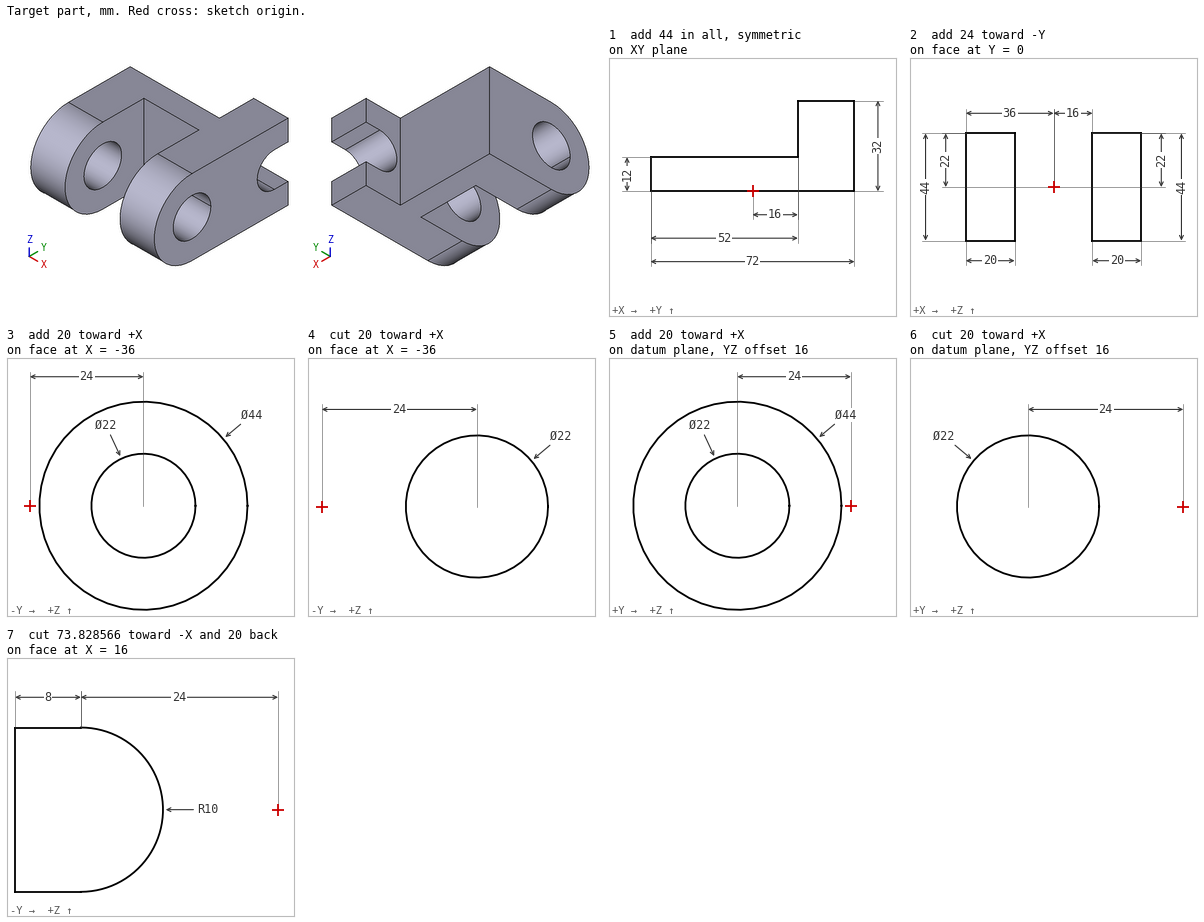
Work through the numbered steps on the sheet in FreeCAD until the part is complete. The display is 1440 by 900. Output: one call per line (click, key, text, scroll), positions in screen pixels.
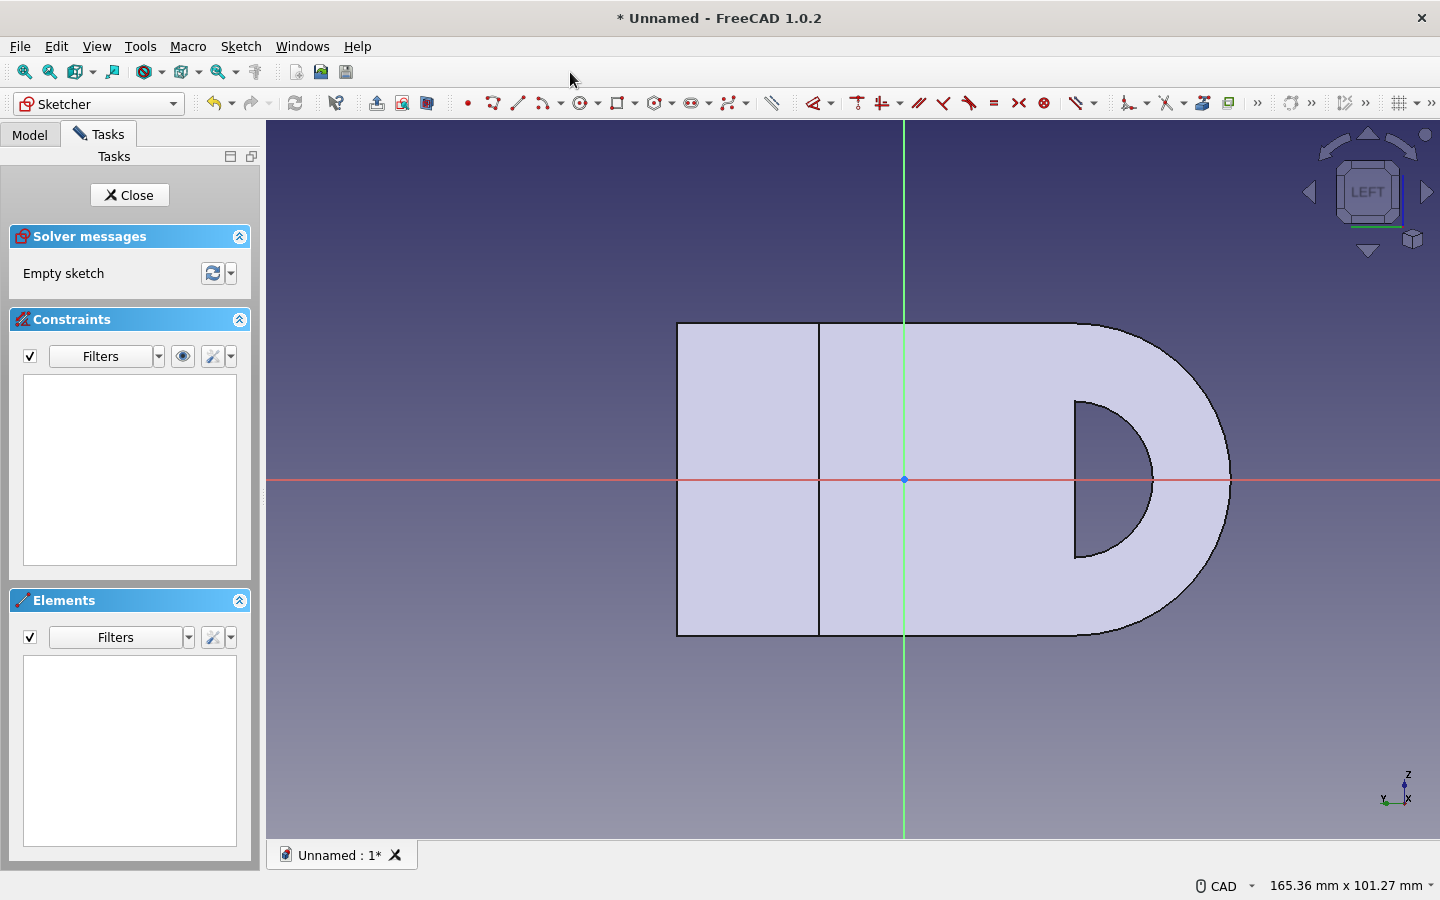
scroll(1171, 480, up, 5)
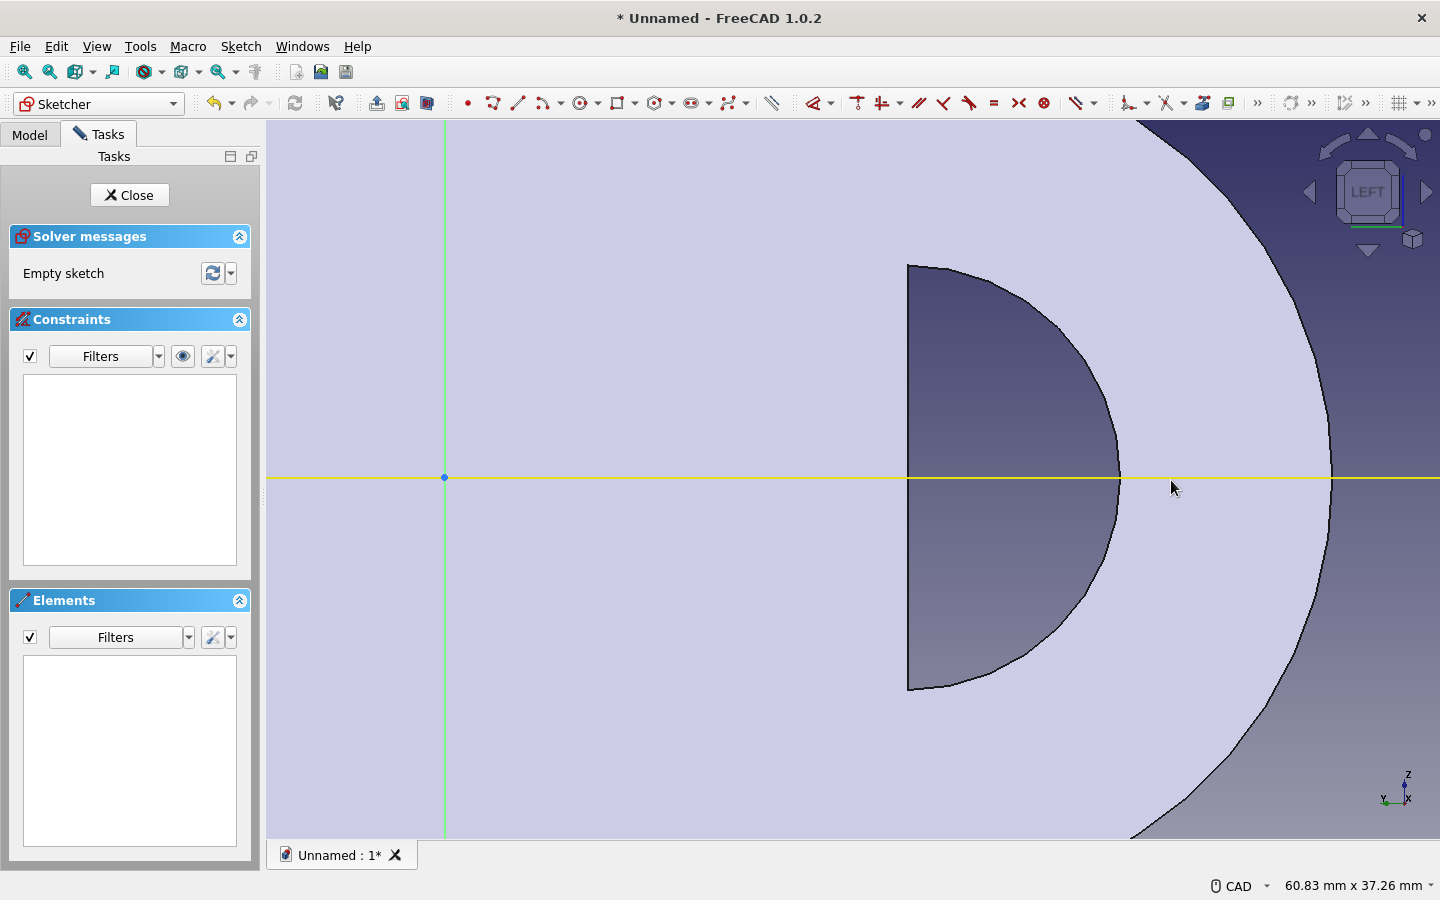
click(580, 104)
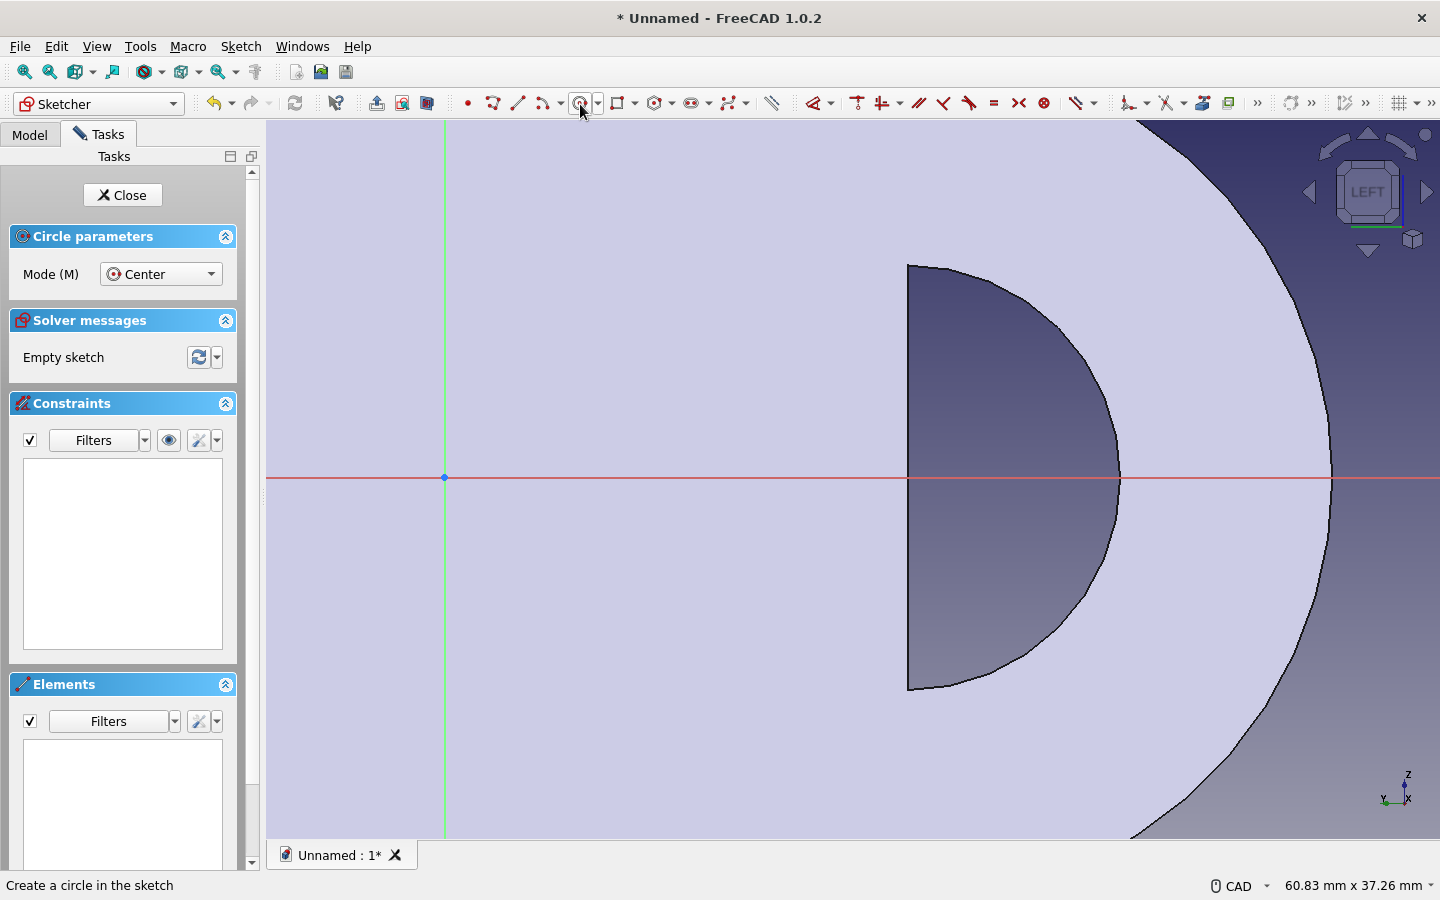
click(908, 478)
click(1058, 328)
key(Escape)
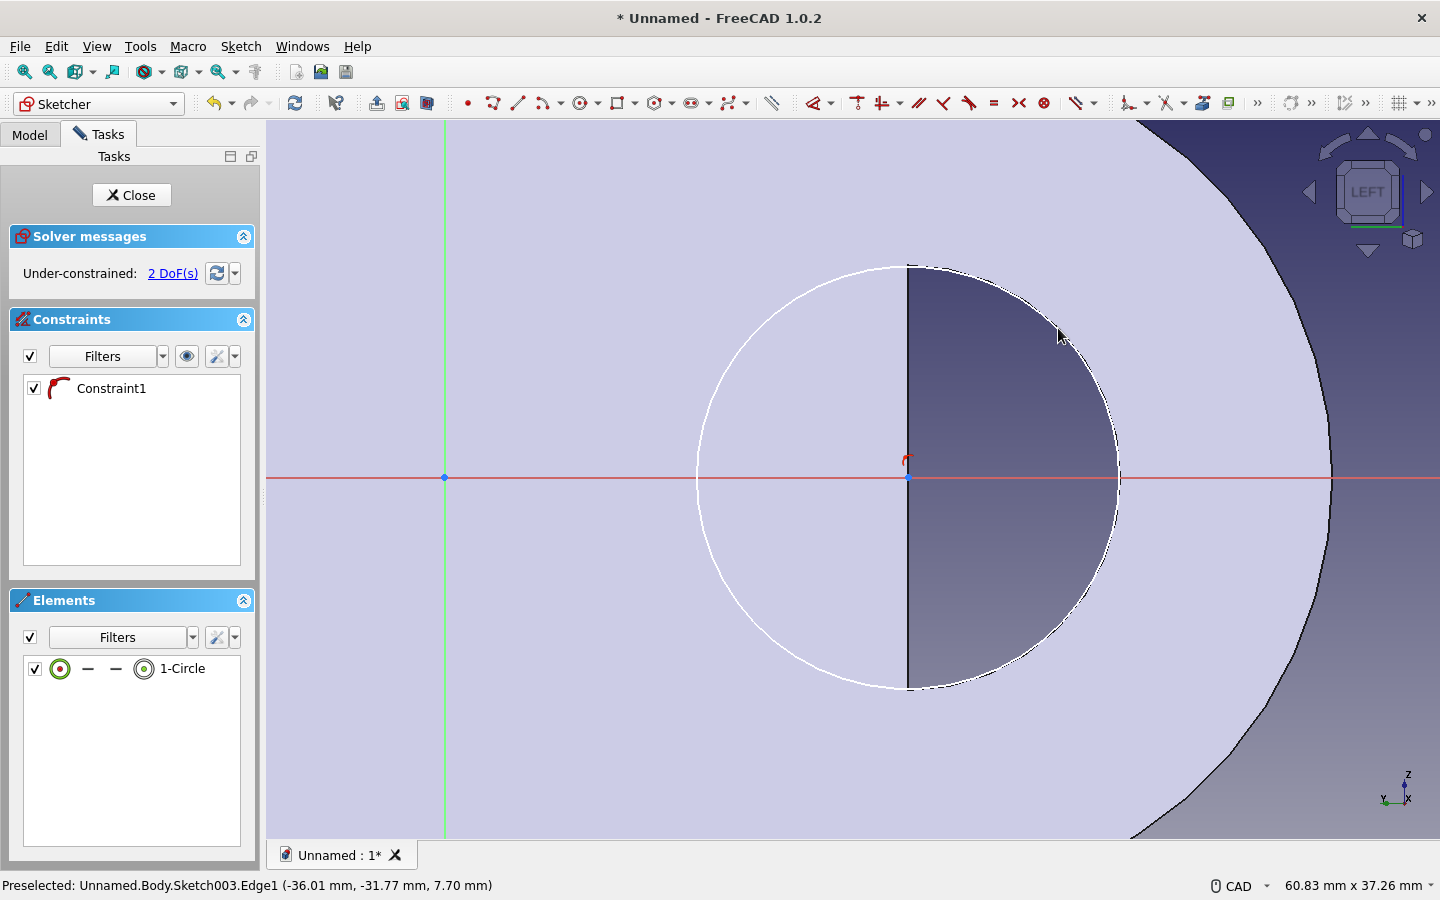
click(812, 104)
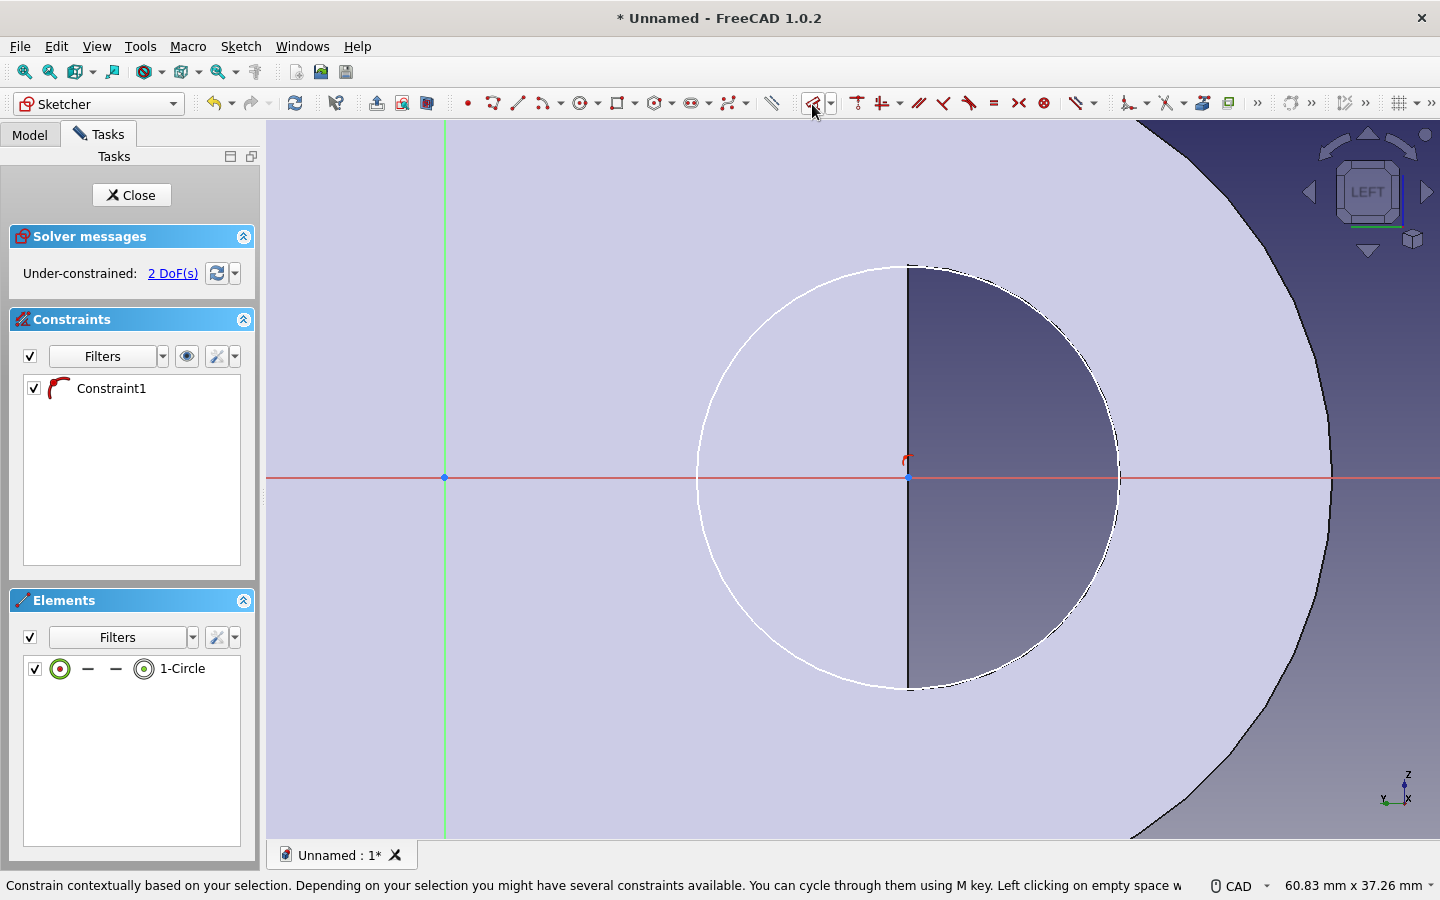
click(1057, 328)
click(1080, 305)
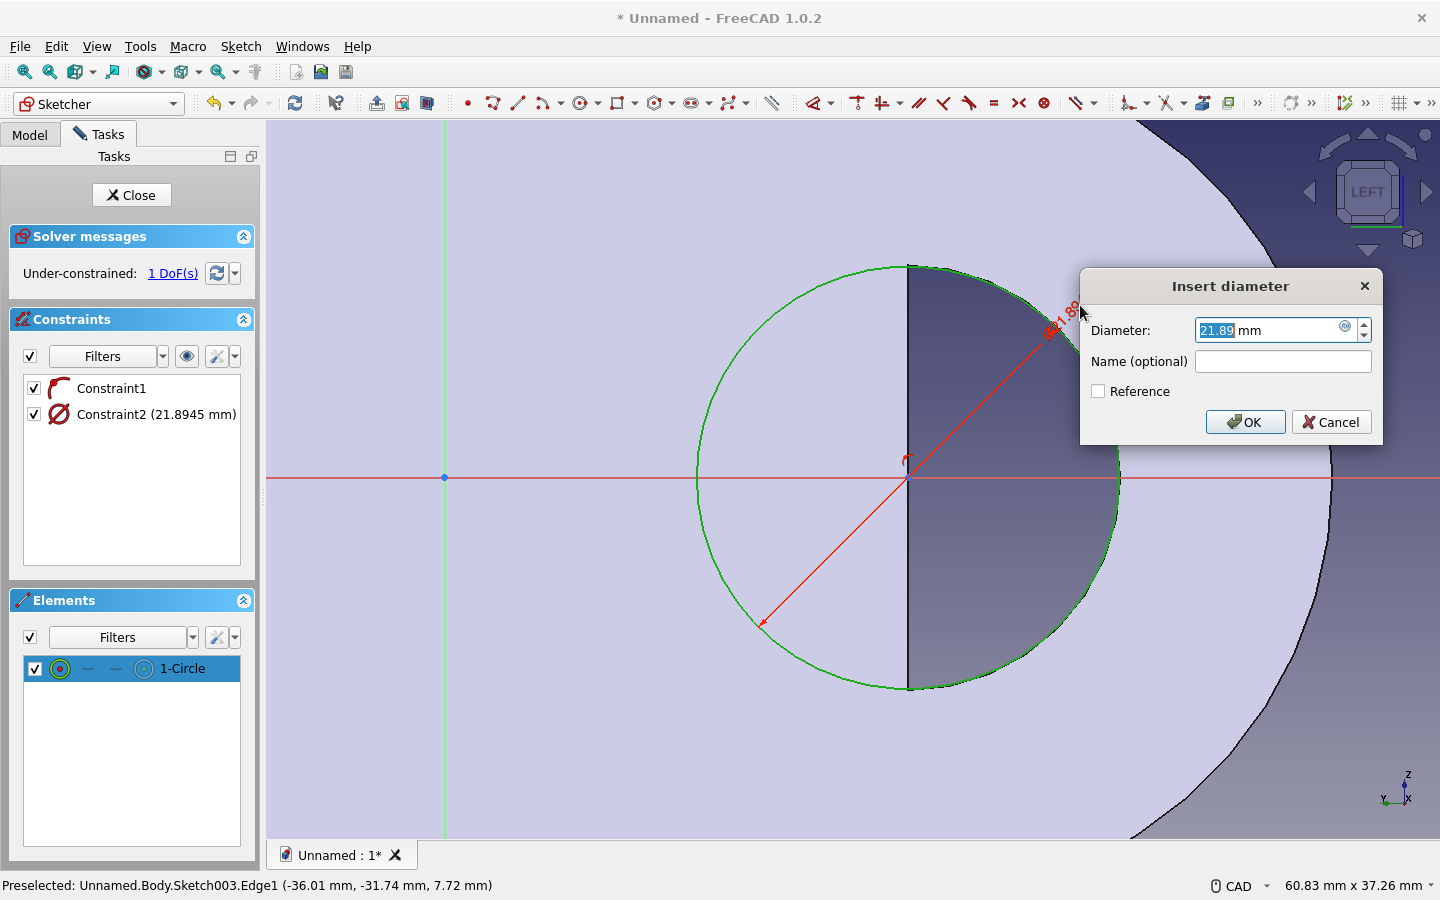
text(22)
key(Return)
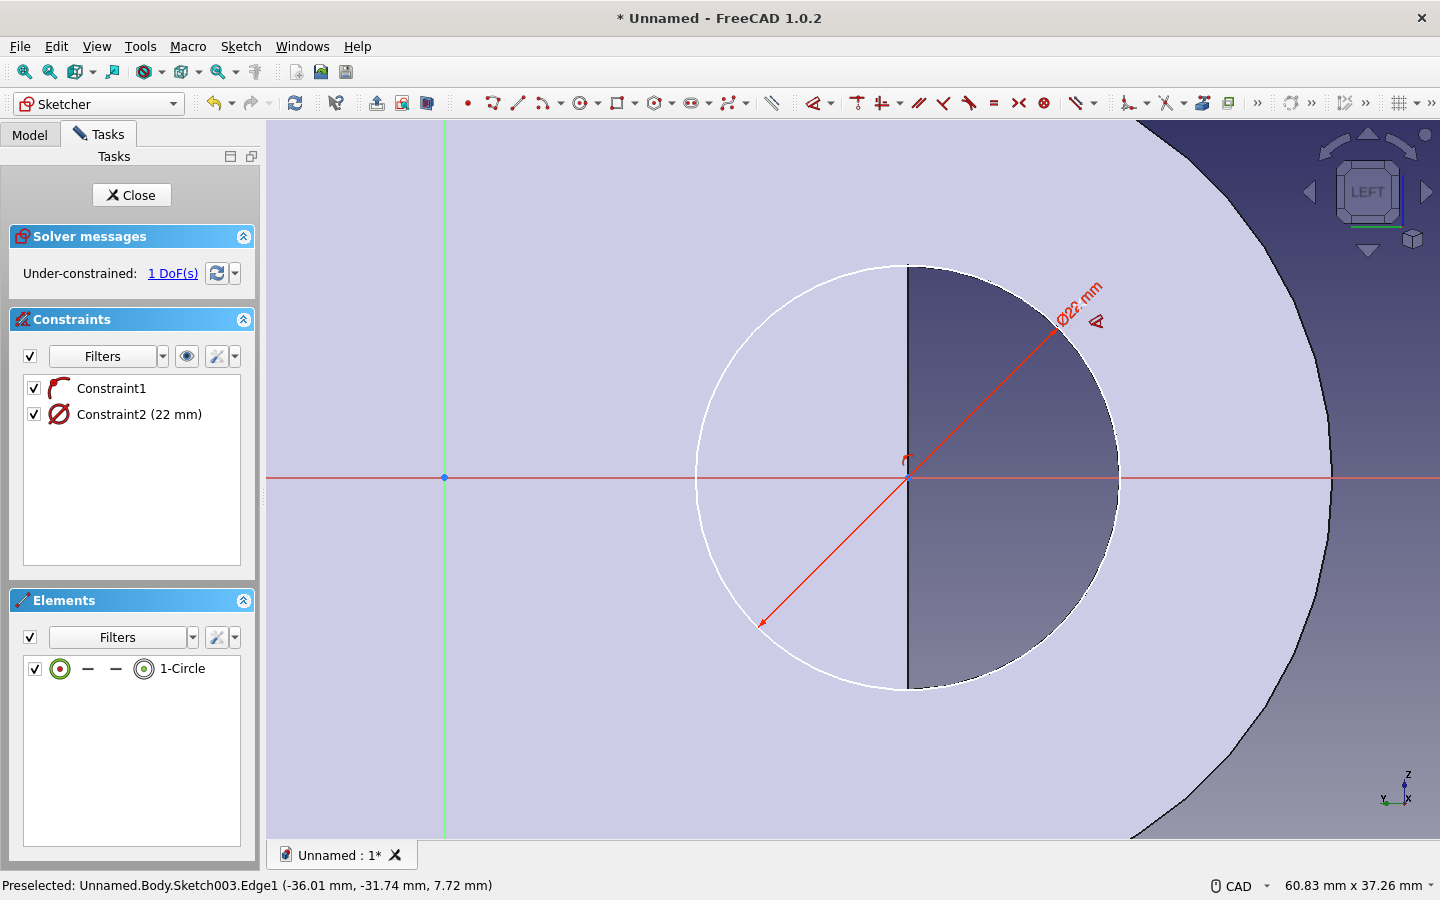
click(908, 478)
click(676, 512)